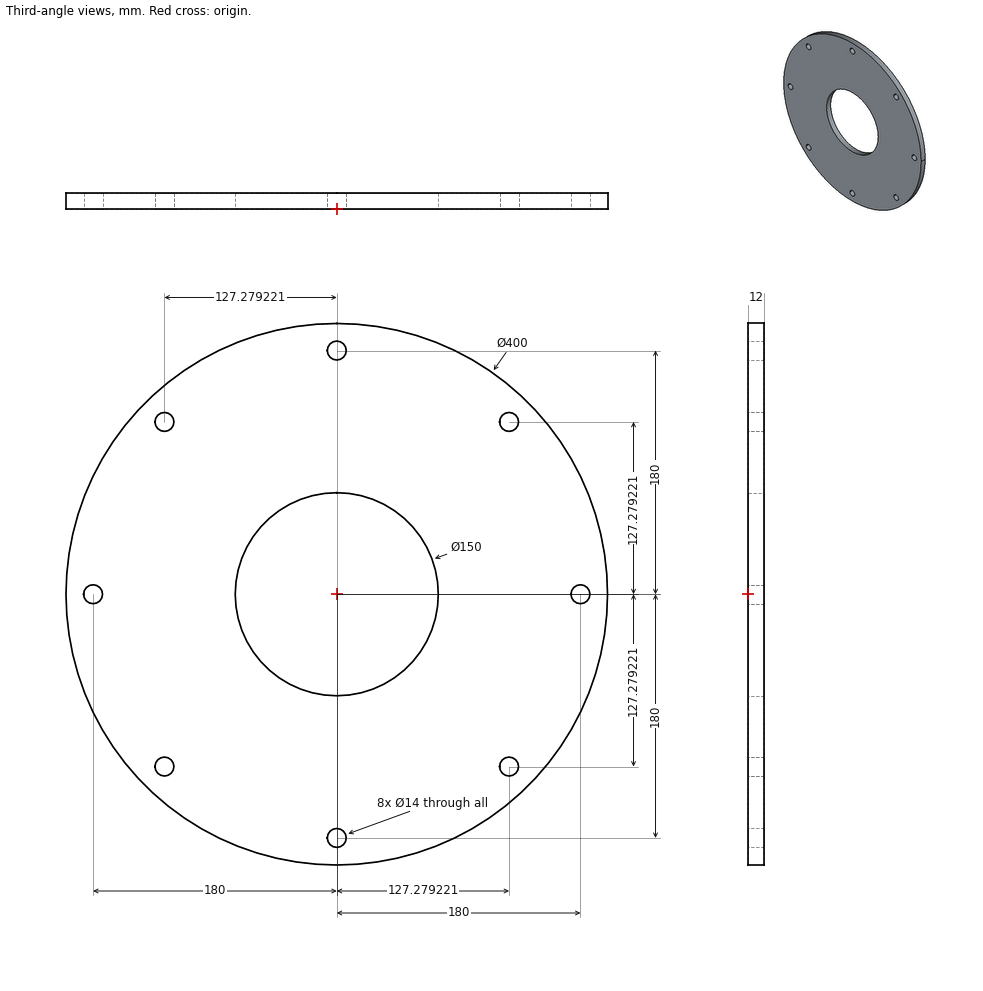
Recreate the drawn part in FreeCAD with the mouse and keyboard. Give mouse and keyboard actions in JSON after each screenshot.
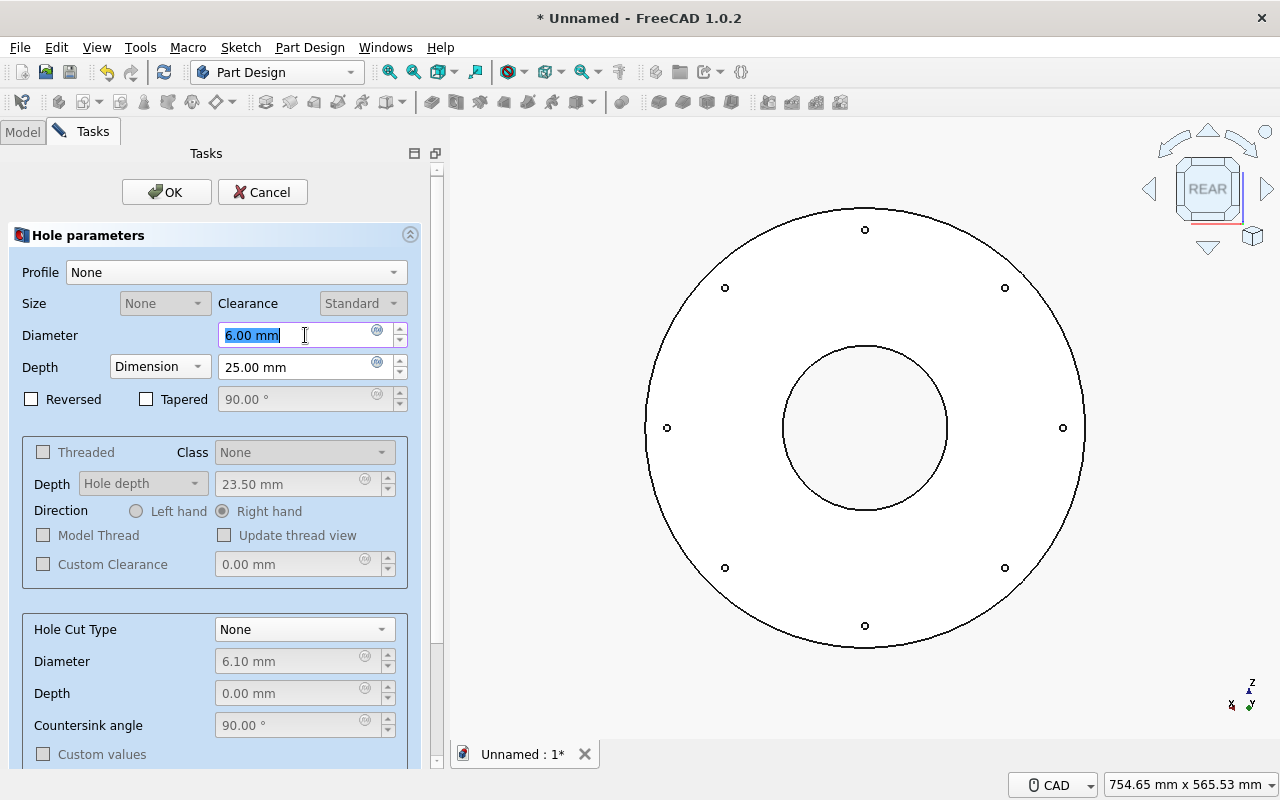
{"action": "type", "text": "14"}
{"action": "key", "text": "Tab"}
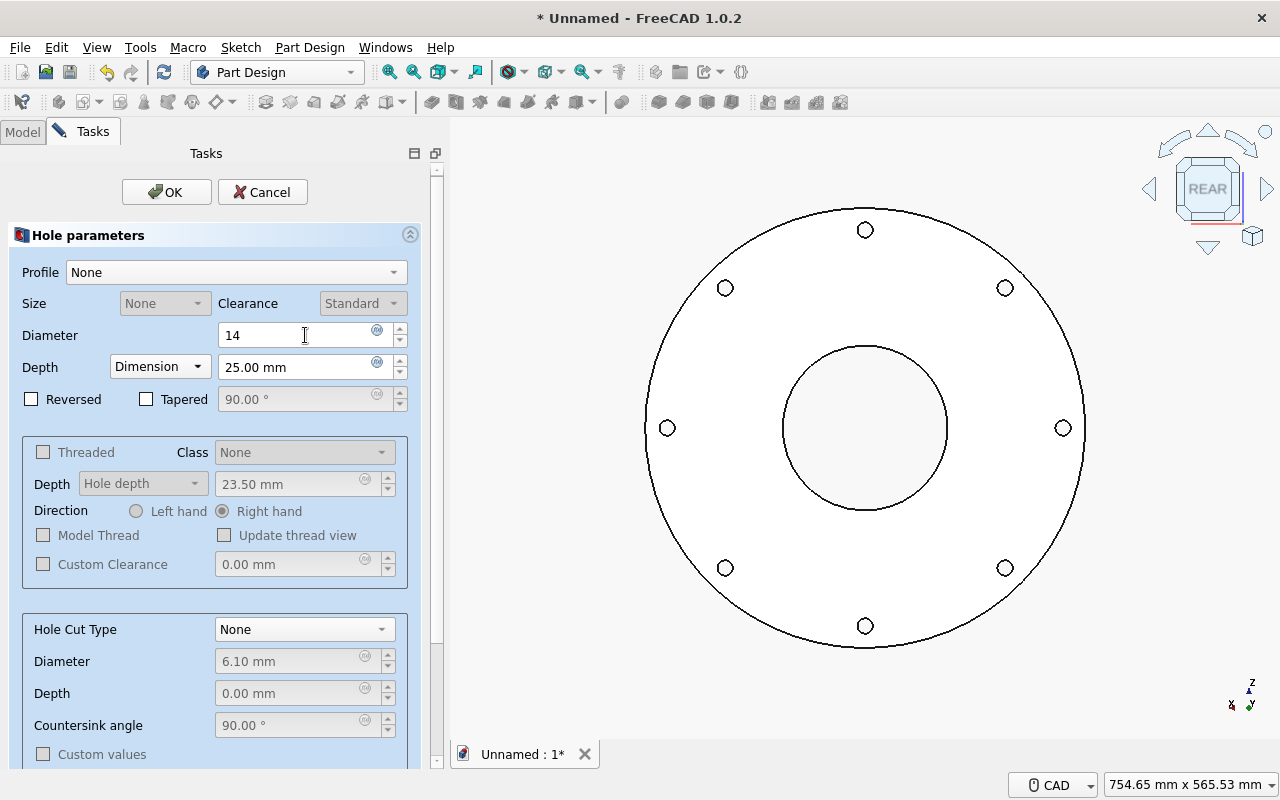
{"action": "left_click", "coordinate": [161, 366]}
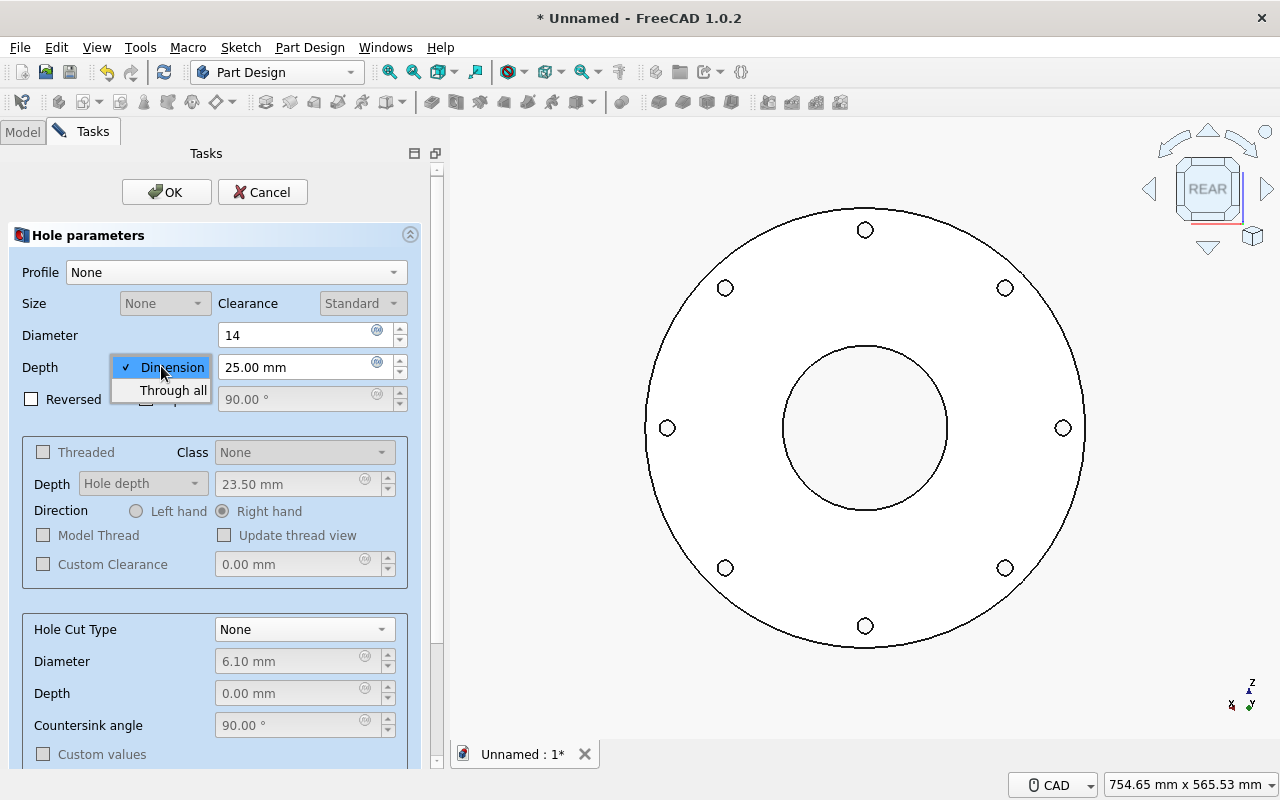
{"action": "left_click", "coordinate": [160, 390]}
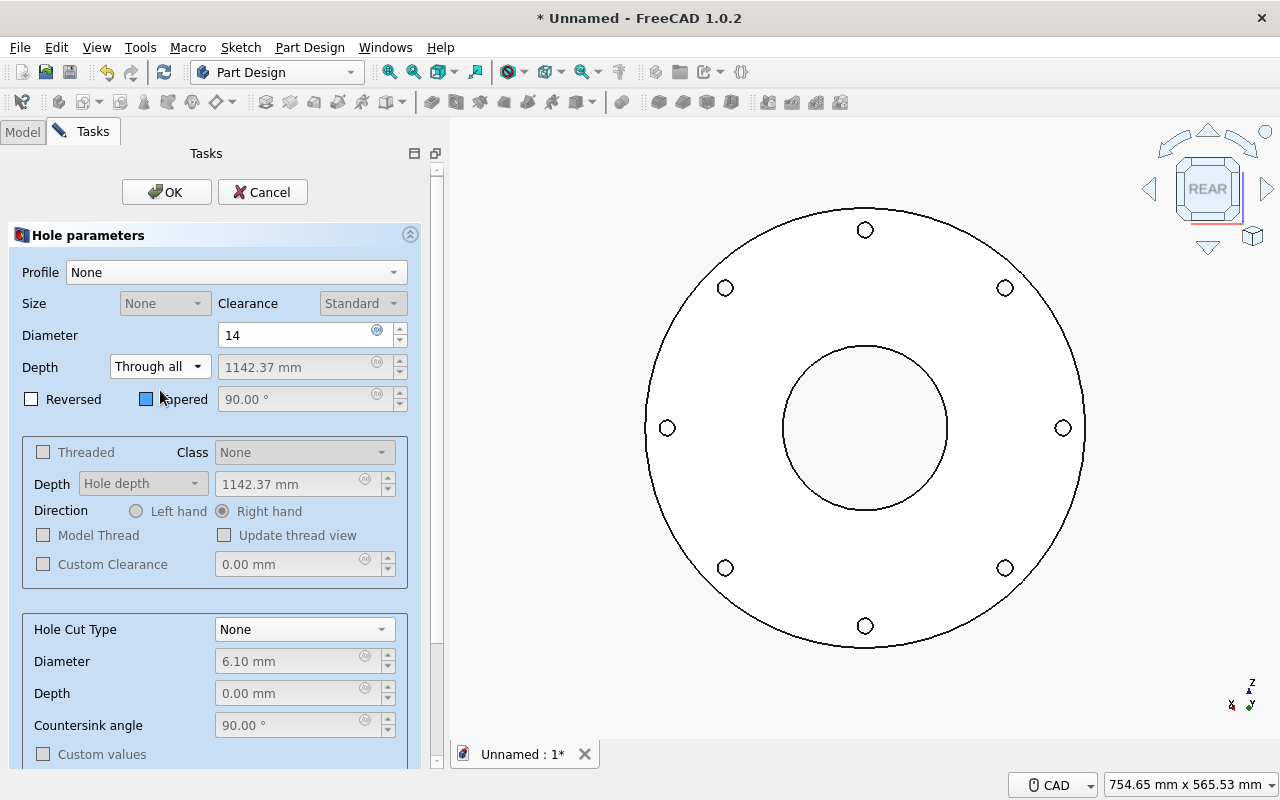
{"action": "left_click", "coordinate": [167, 192]}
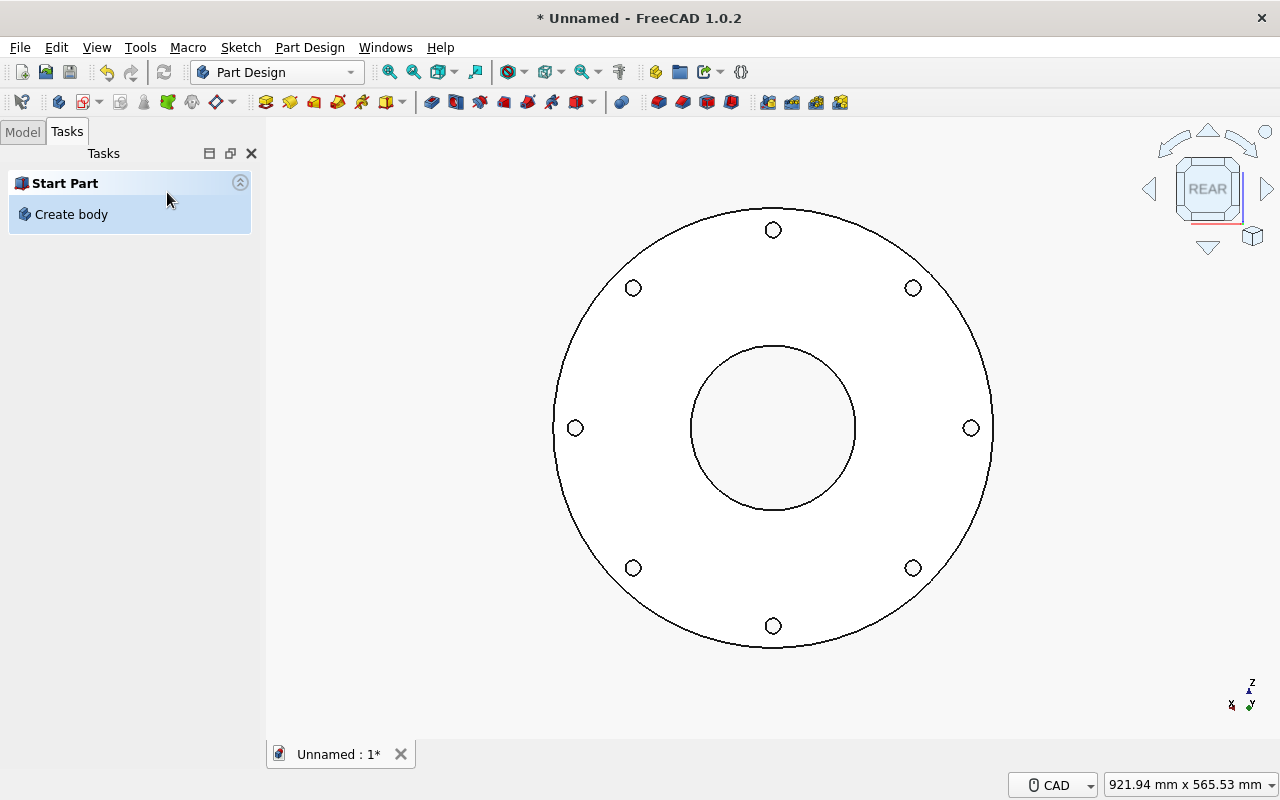
{"action": "key", "text": "0"}